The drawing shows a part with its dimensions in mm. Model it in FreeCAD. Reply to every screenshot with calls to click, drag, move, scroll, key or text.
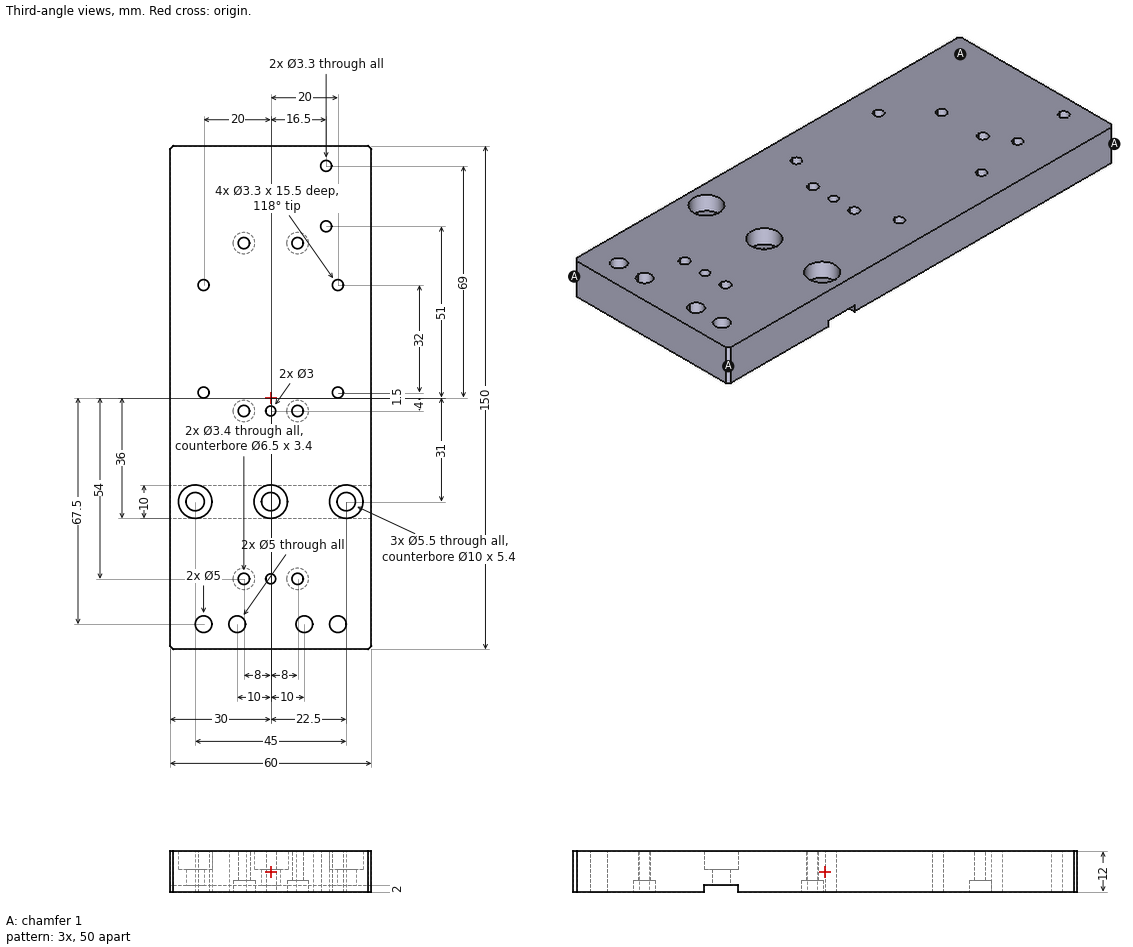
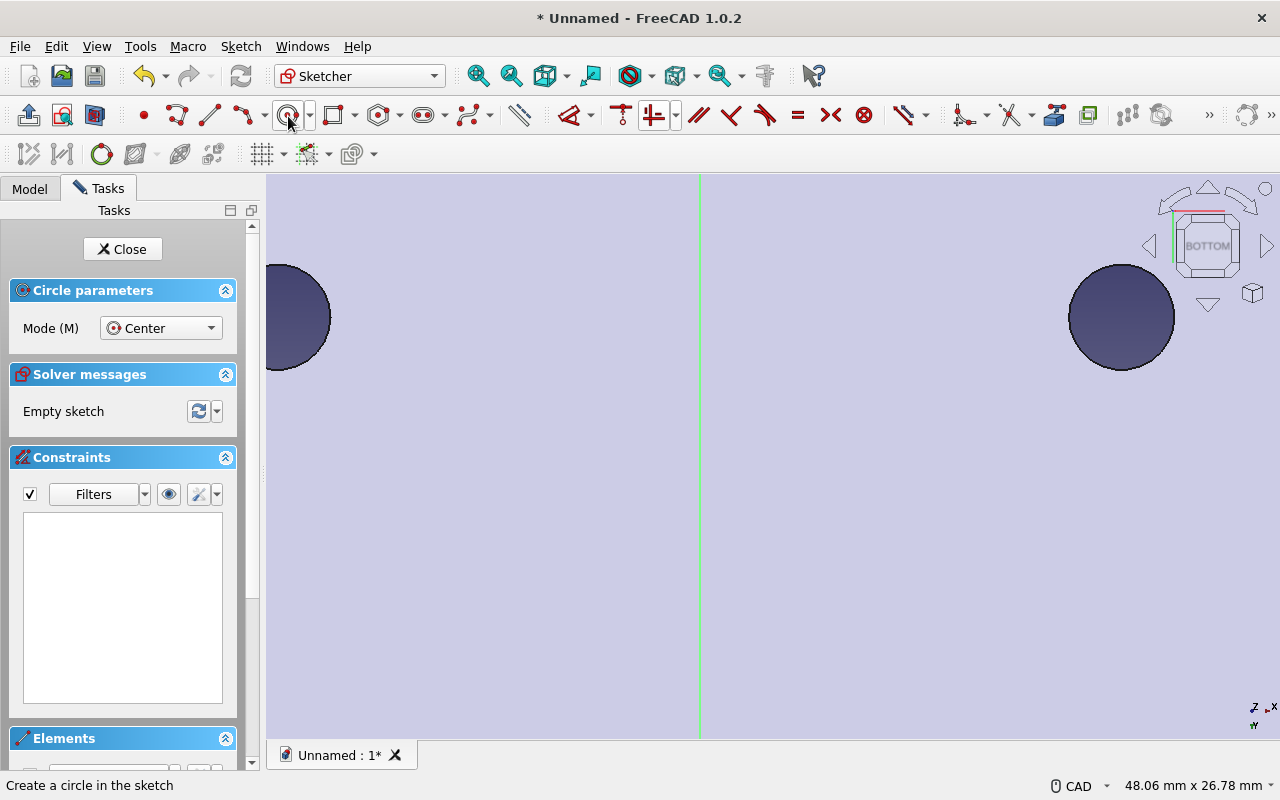
click(489, 317)
click(526, 280)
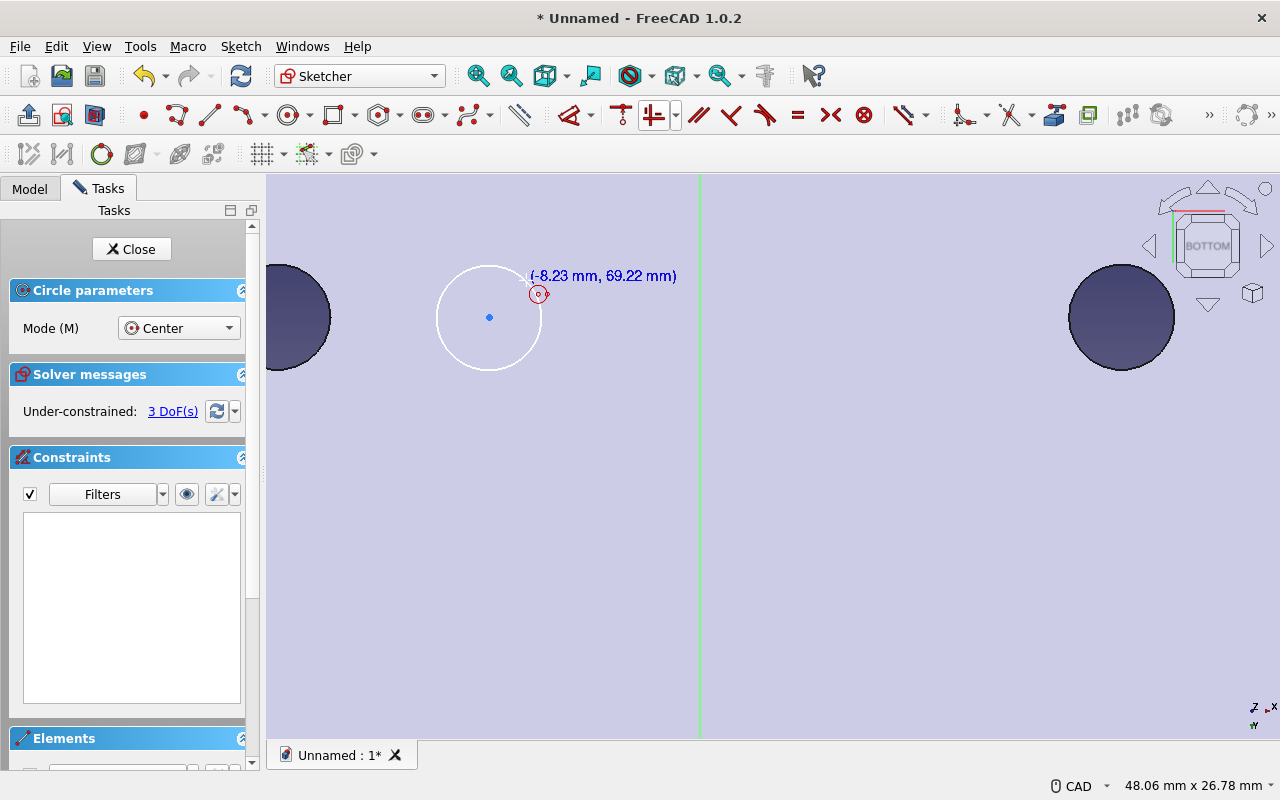
click(911, 317)
click(948, 280)
key(Escape)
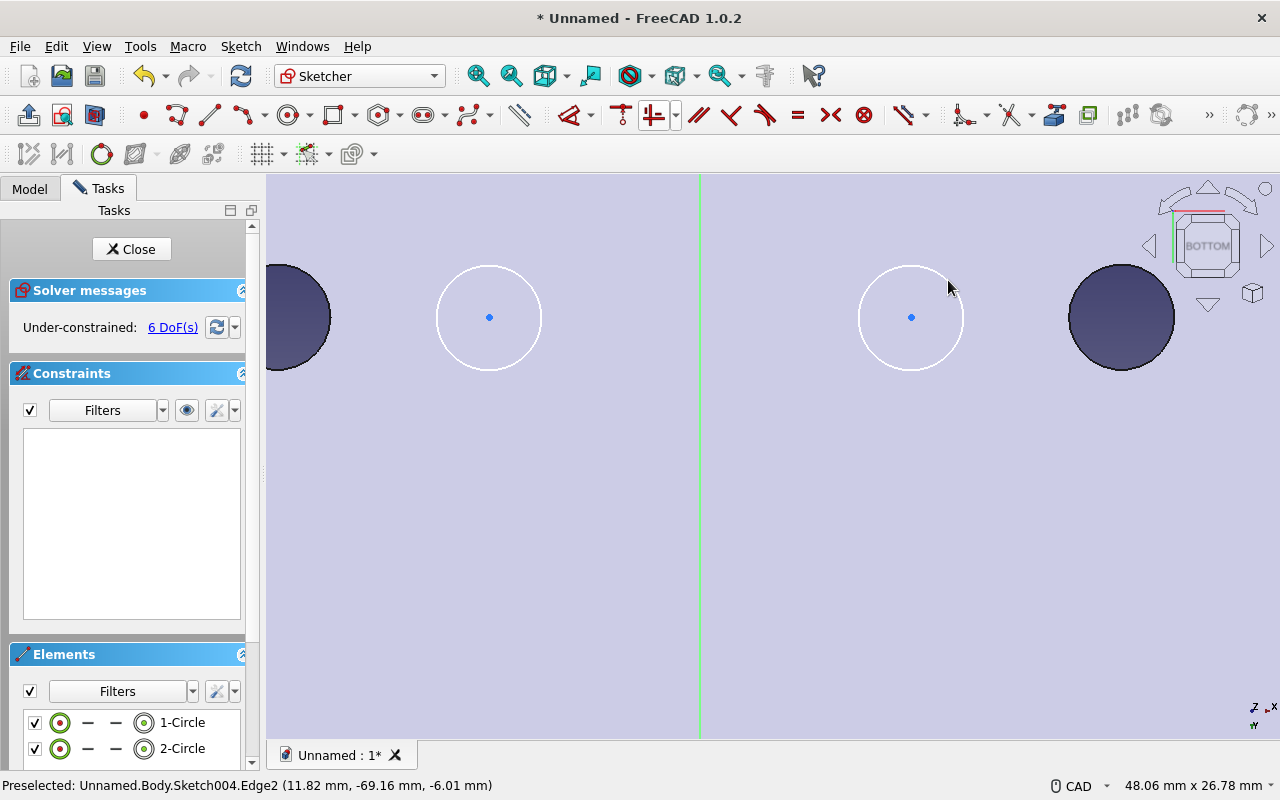
click(526, 281)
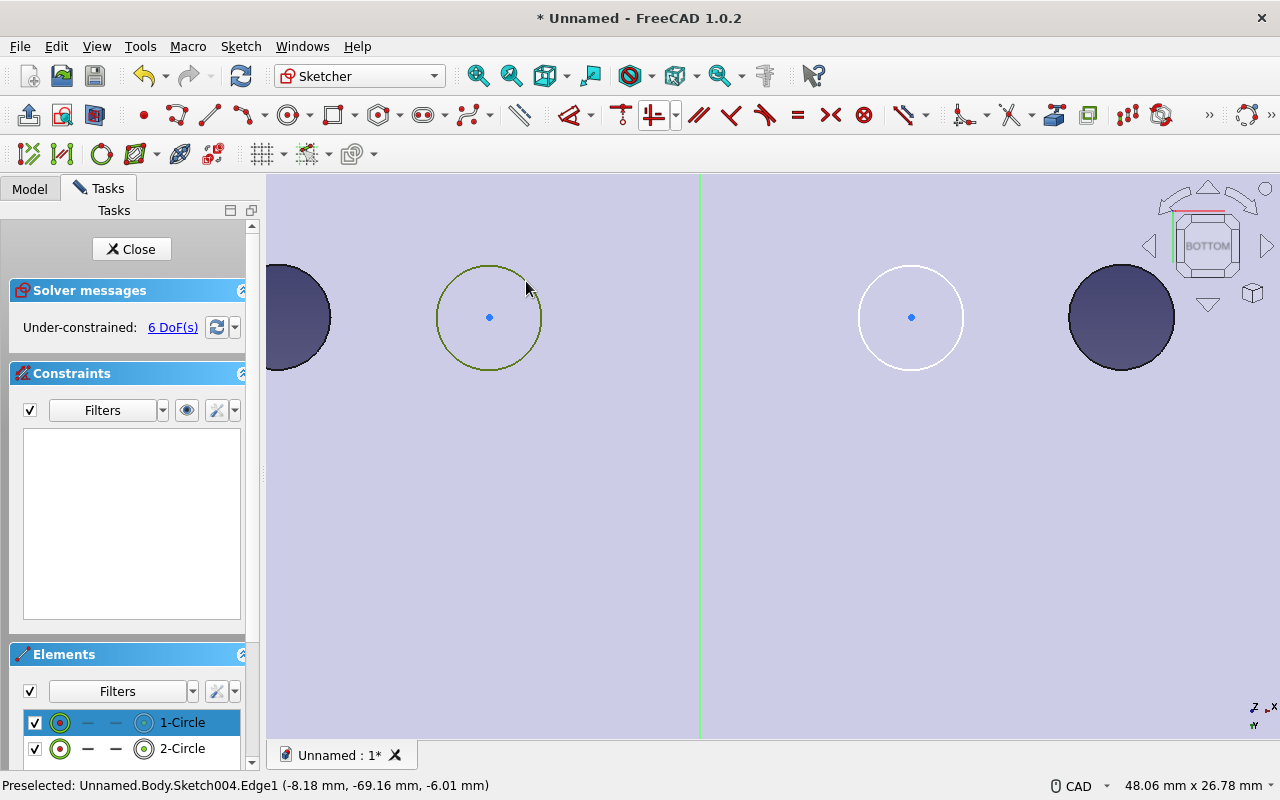
click(948, 281)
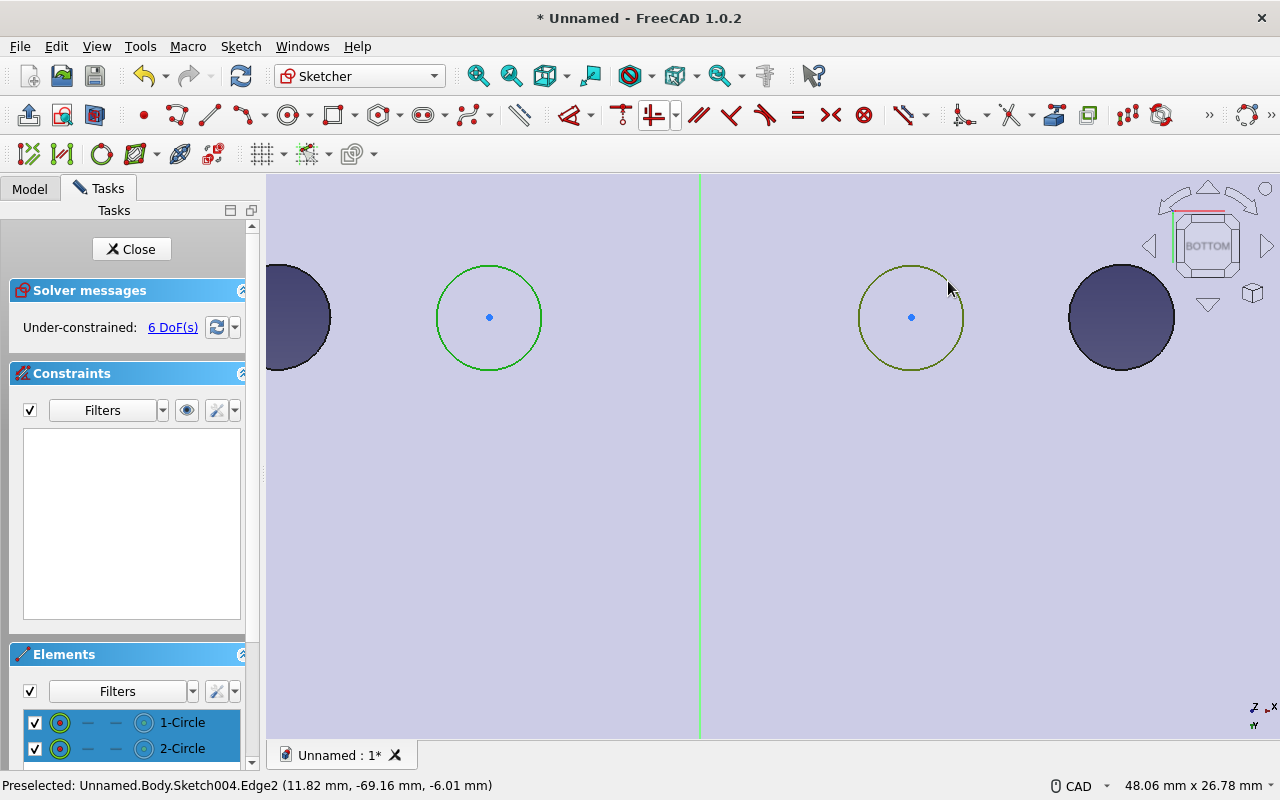
click(798, 116)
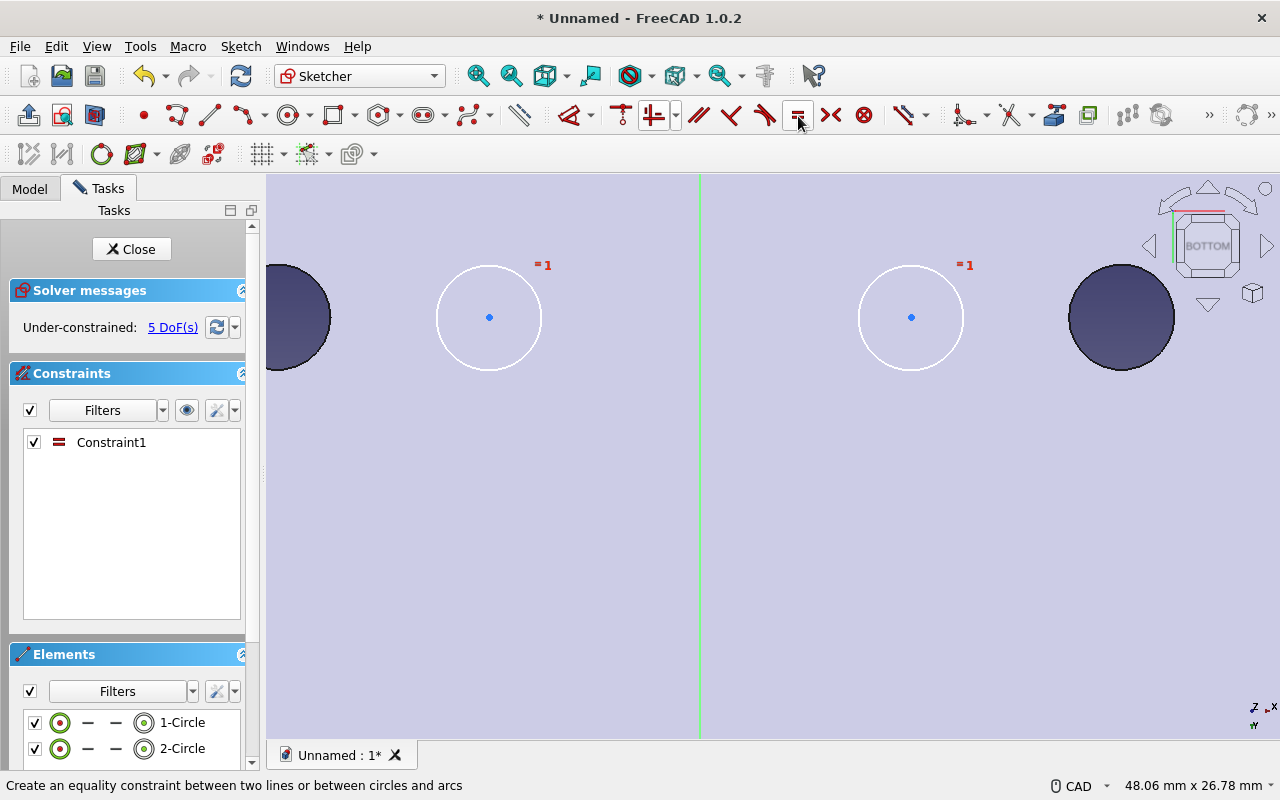
click(489, 318)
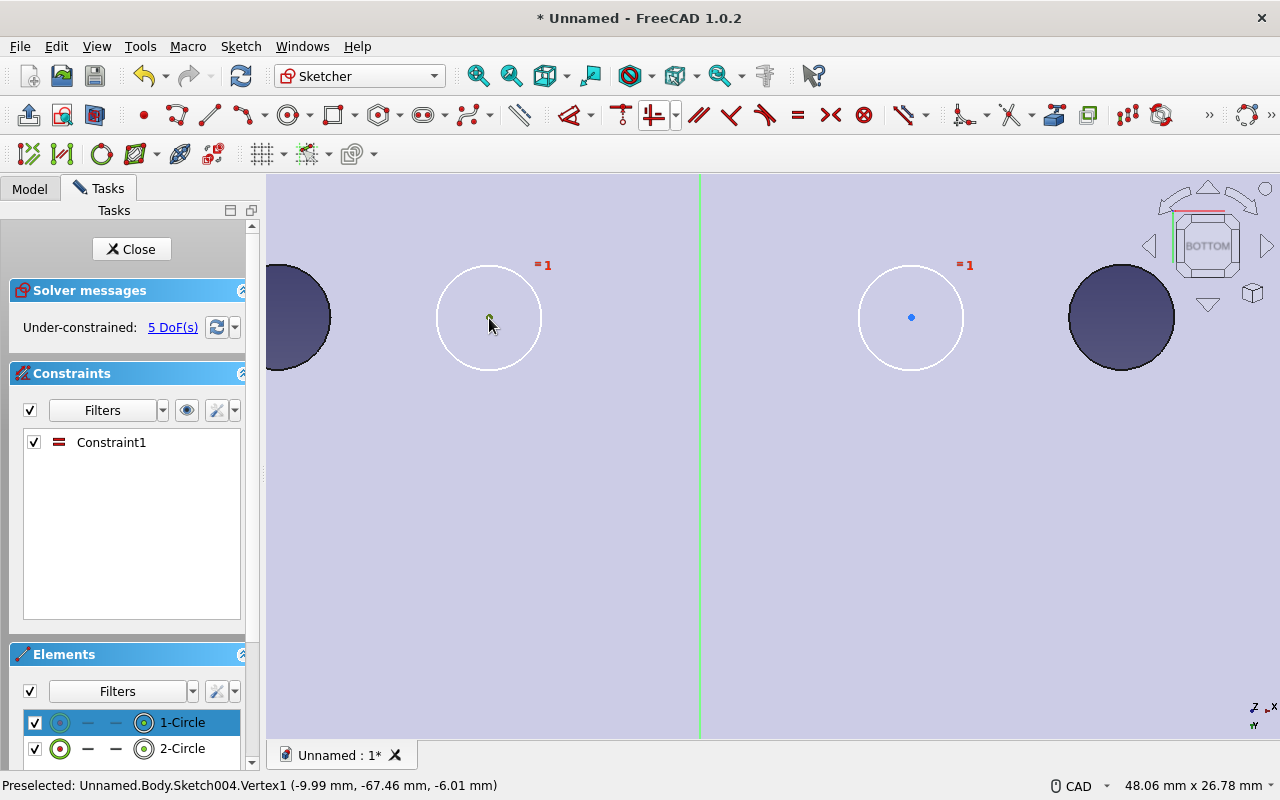
click(911, 318)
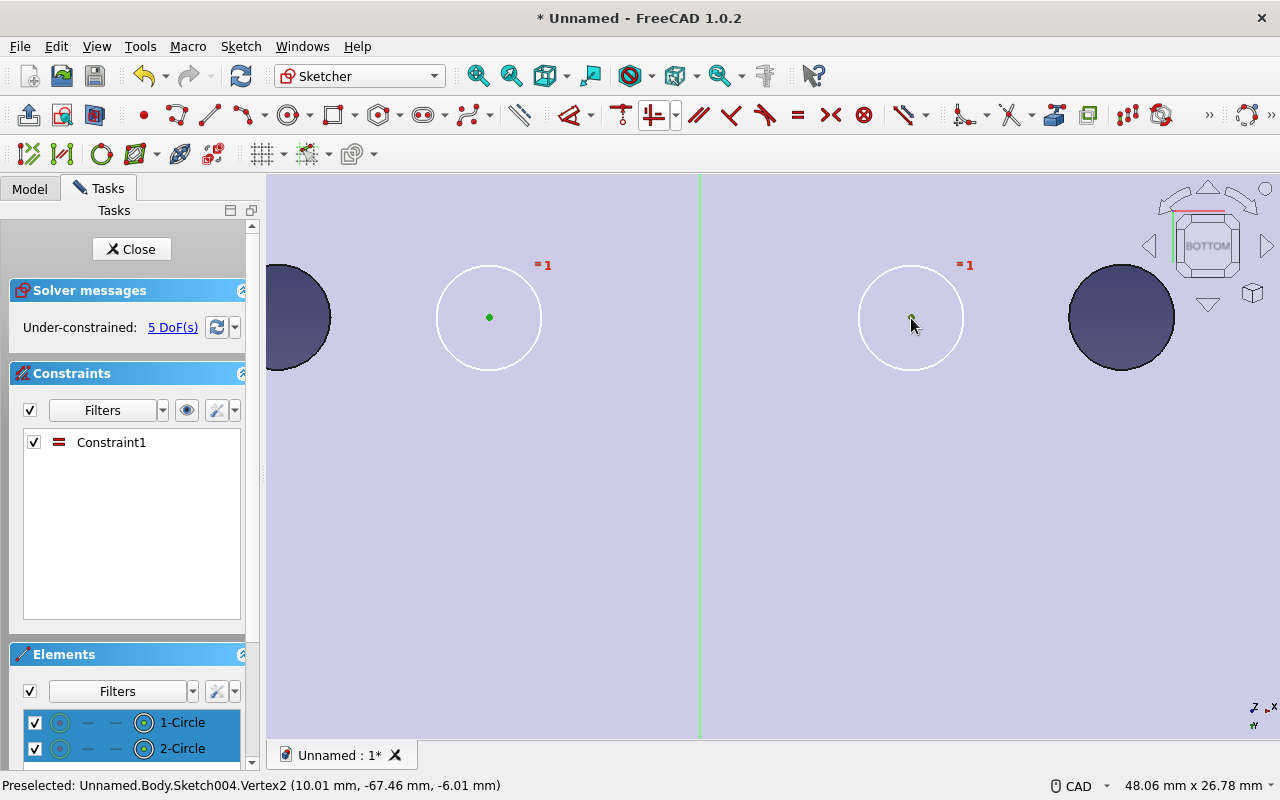
key(h)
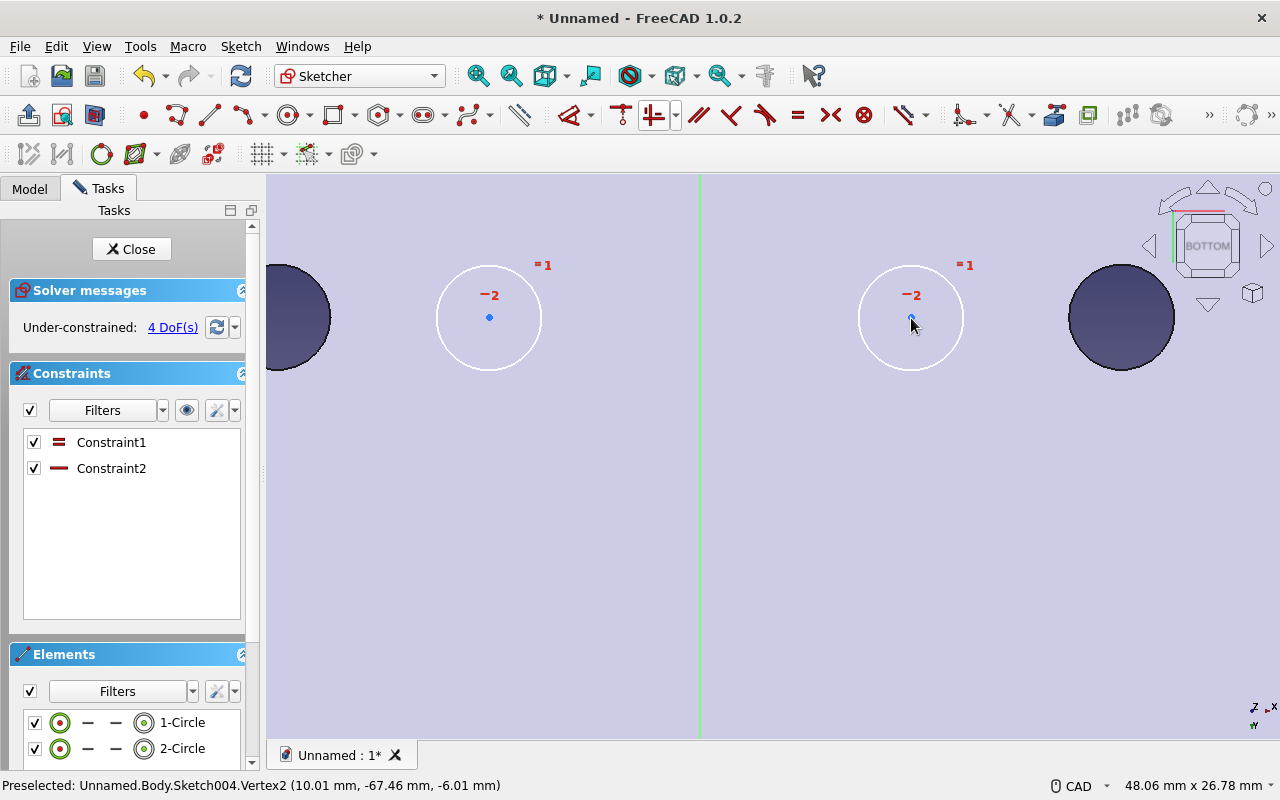
click(568, 116)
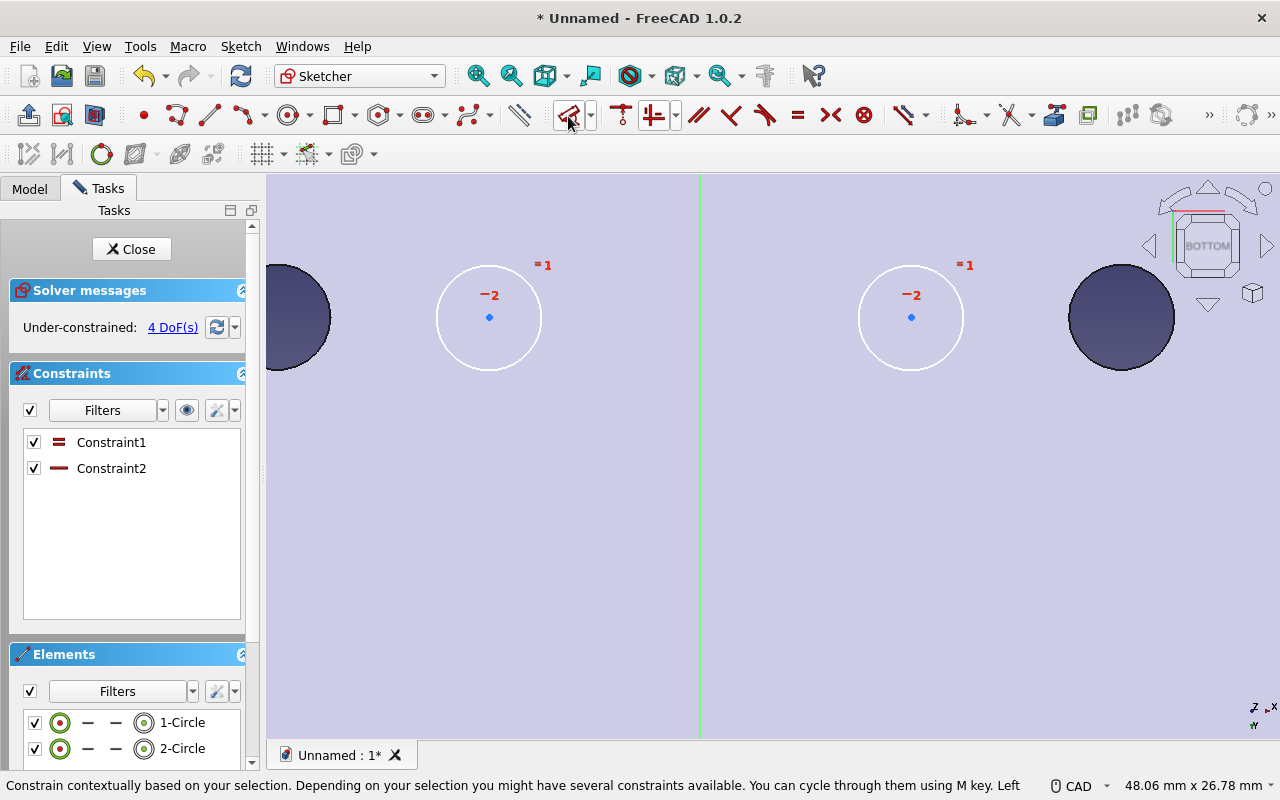
click(526, 281)
click(549, 258)